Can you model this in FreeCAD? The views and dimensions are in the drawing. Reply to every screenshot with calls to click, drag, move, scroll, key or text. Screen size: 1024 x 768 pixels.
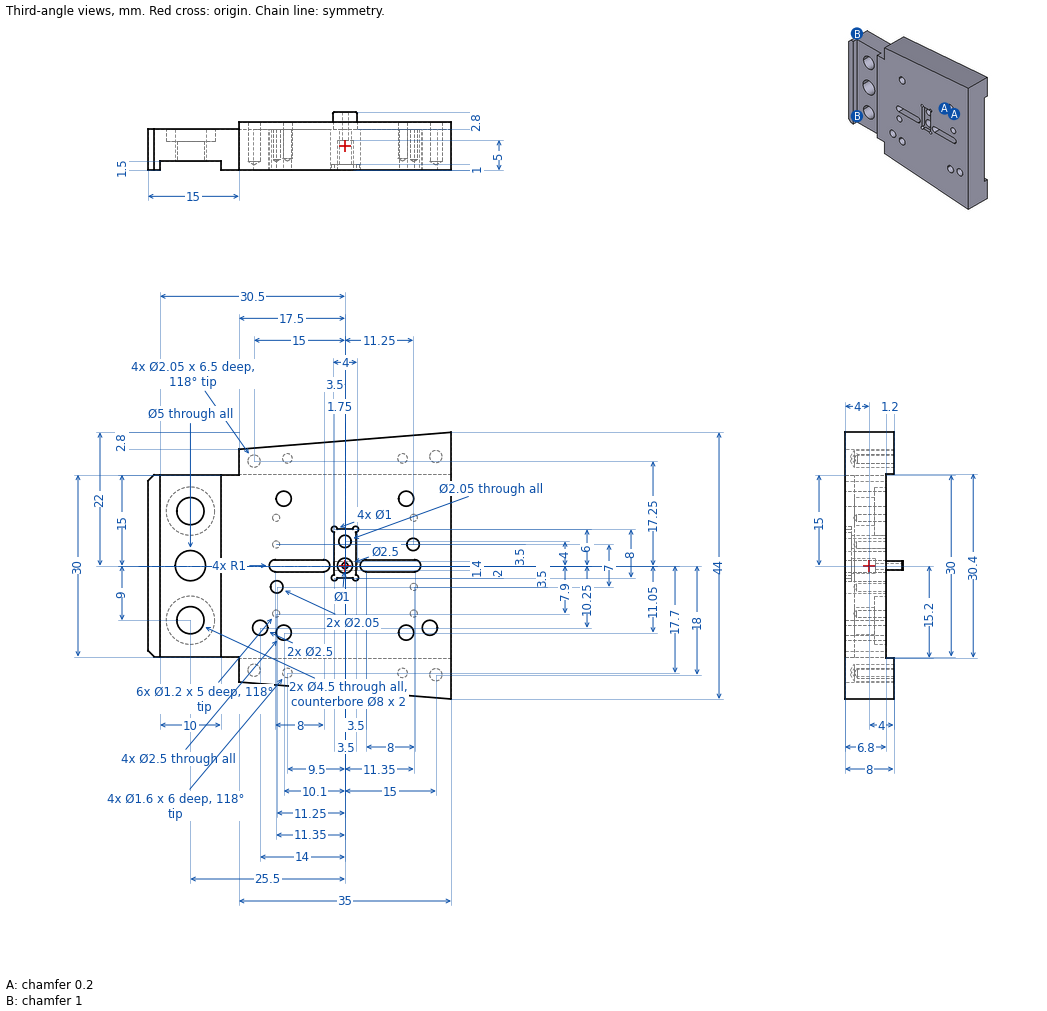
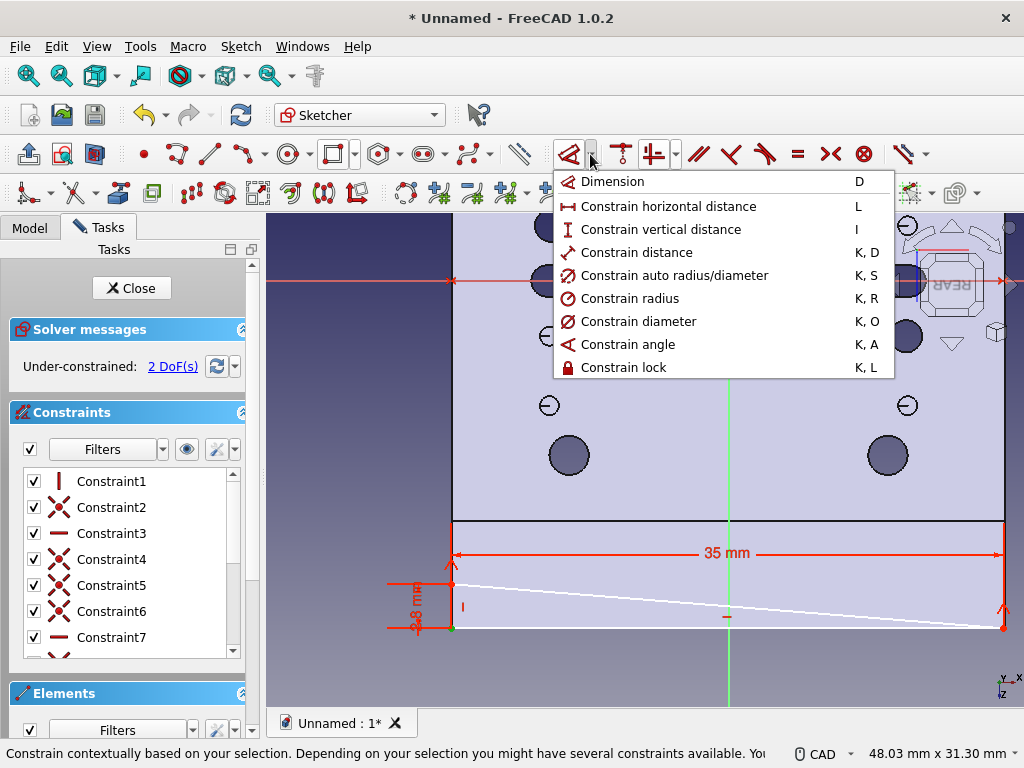
click(724, 230)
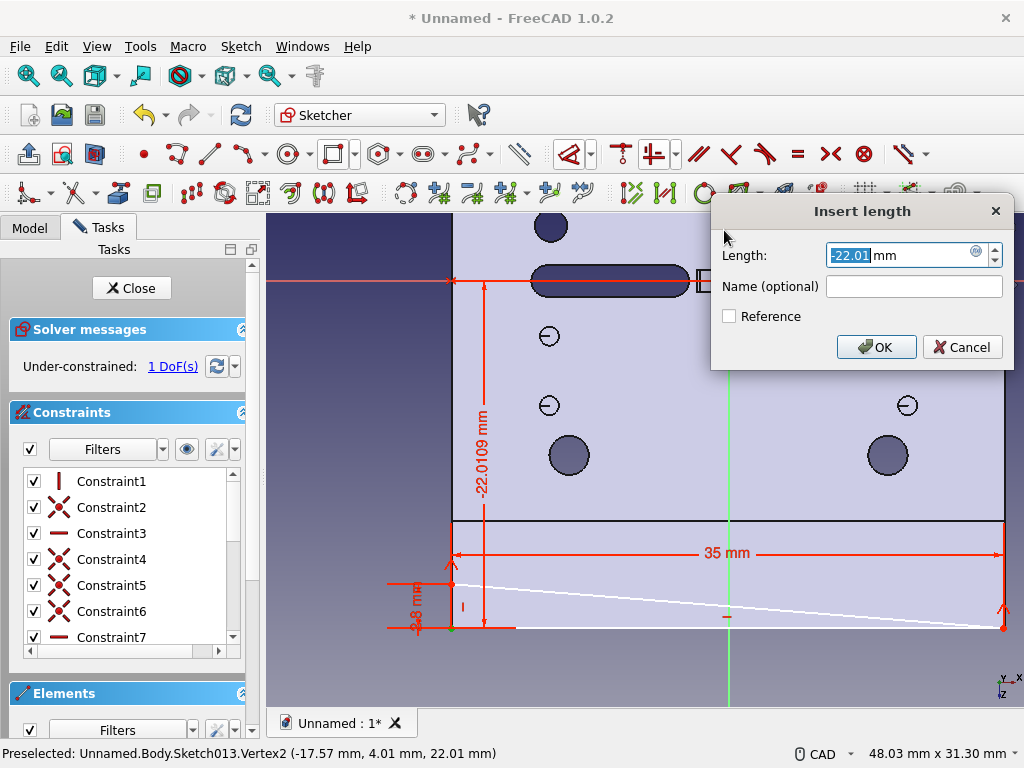
text(-22)
key(Return)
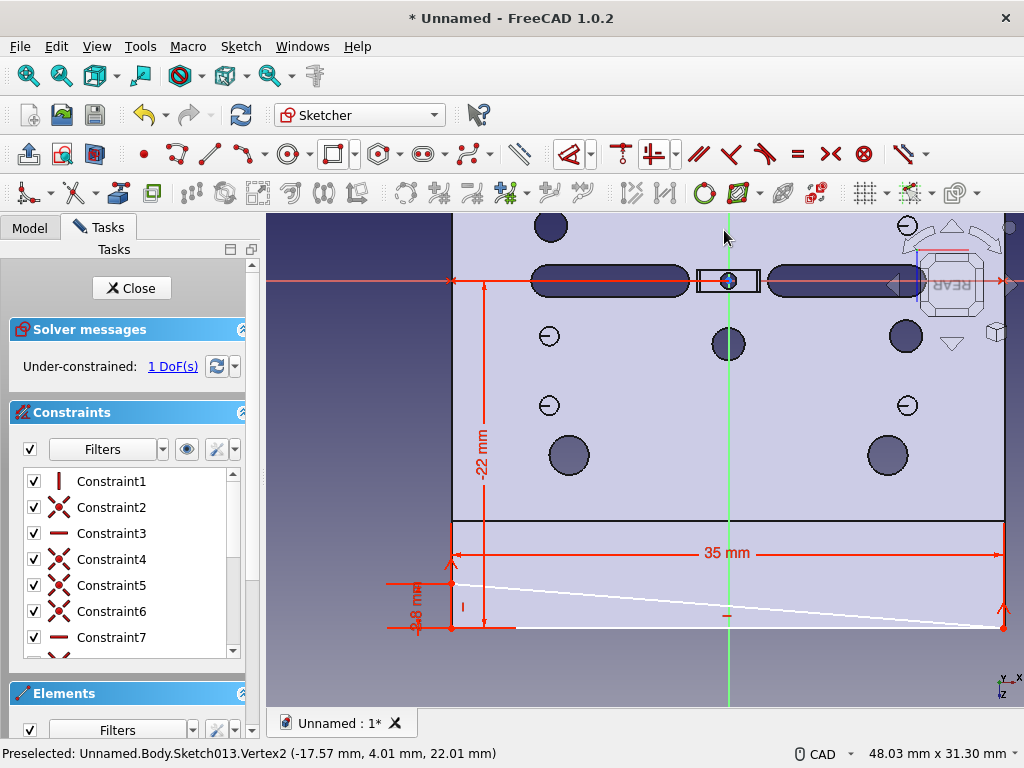
click(451, 584)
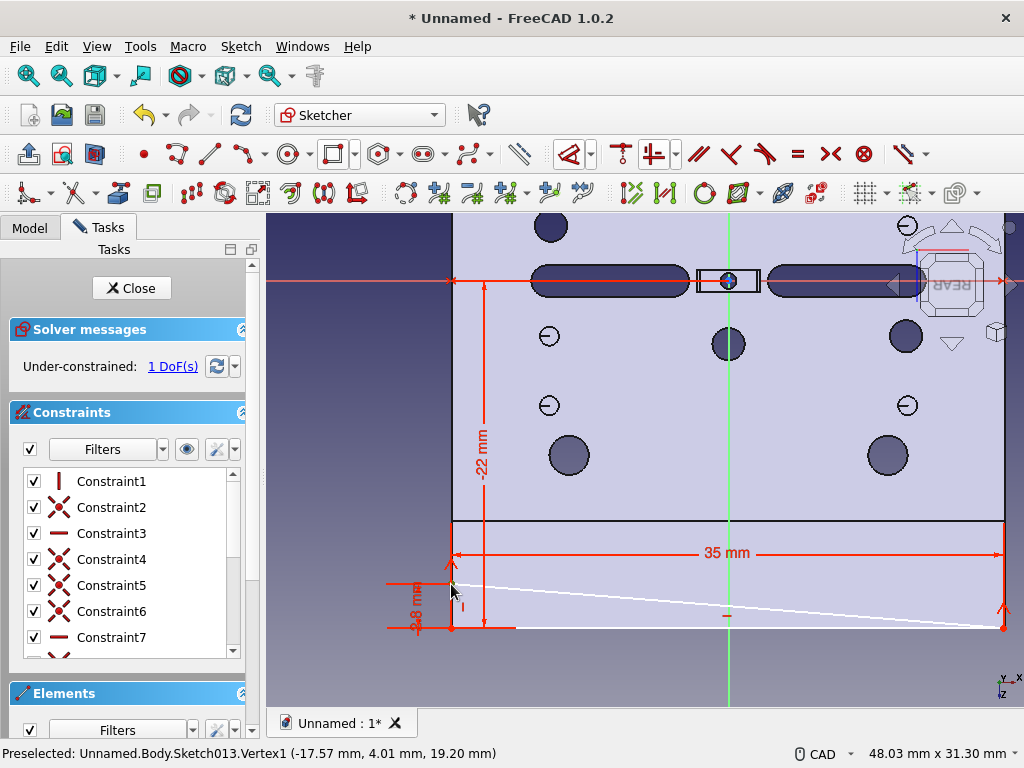
click(590, 154)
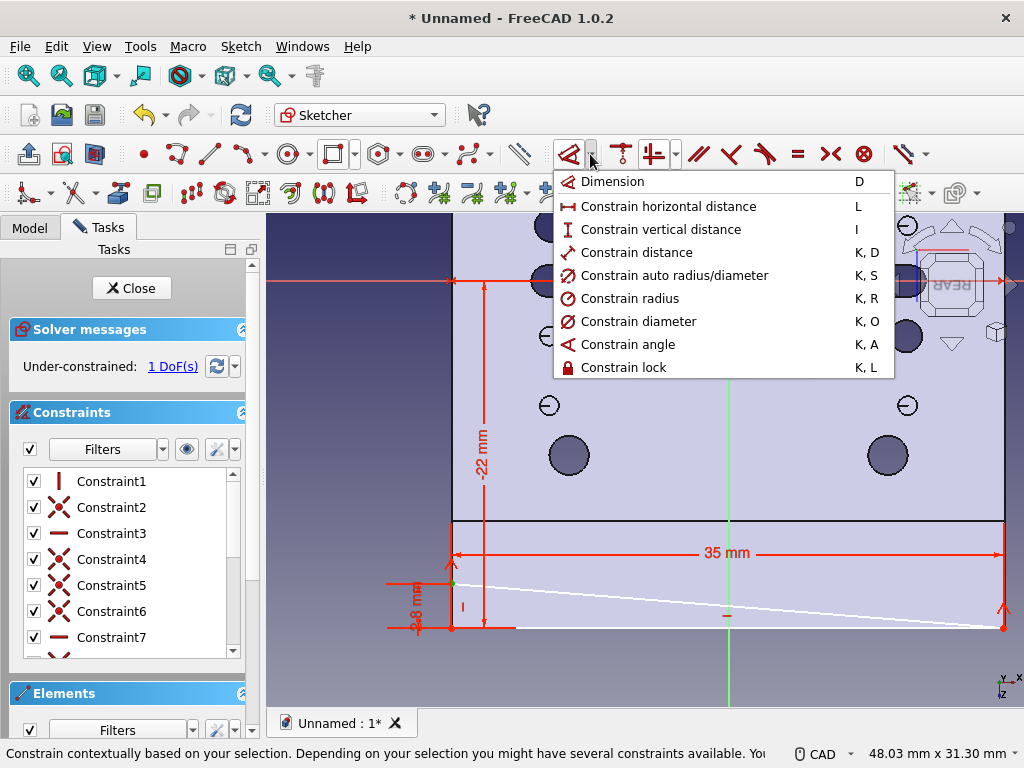
click(724, 206)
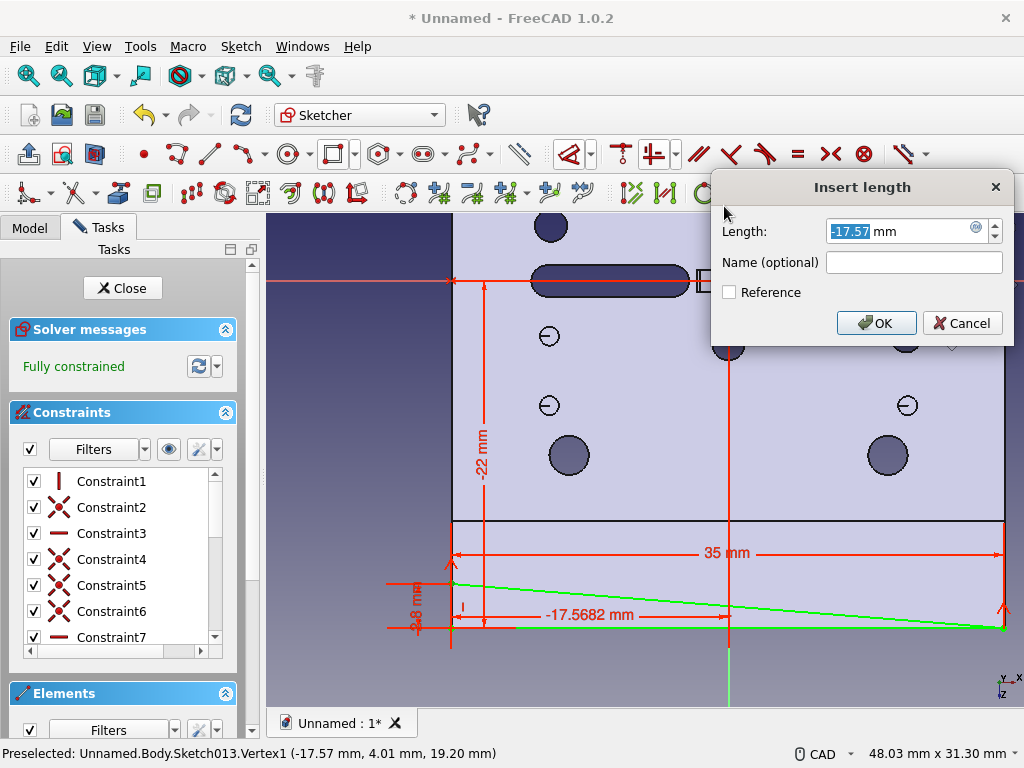
text(-17.5)
key(Return)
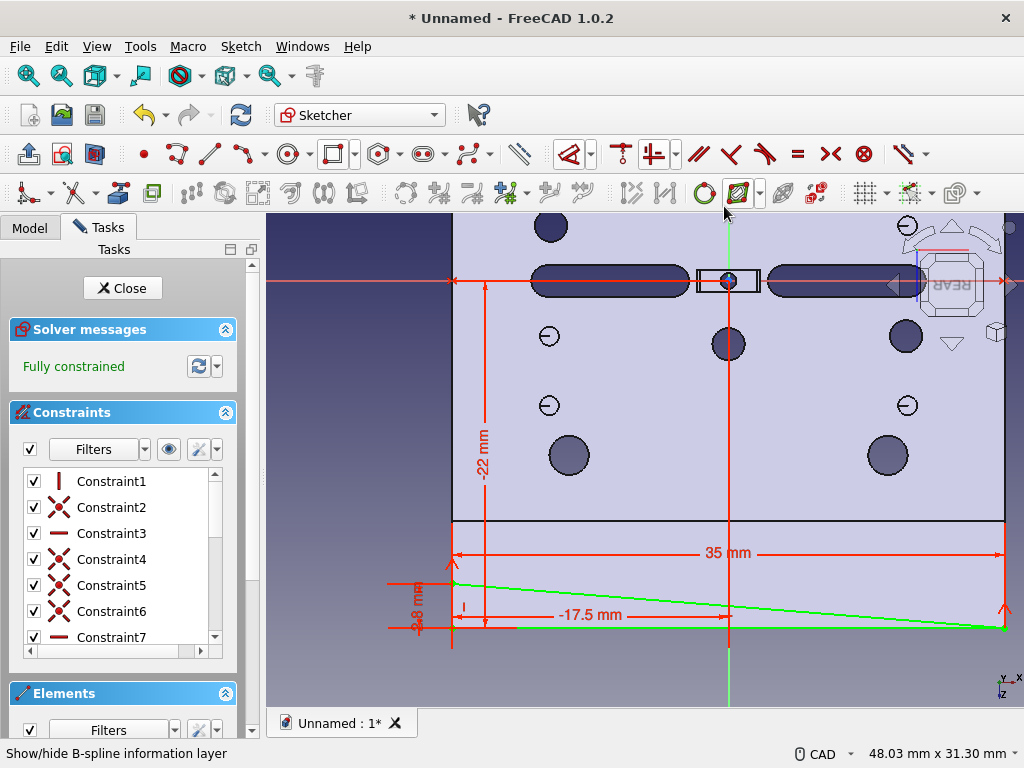
click(123, 288)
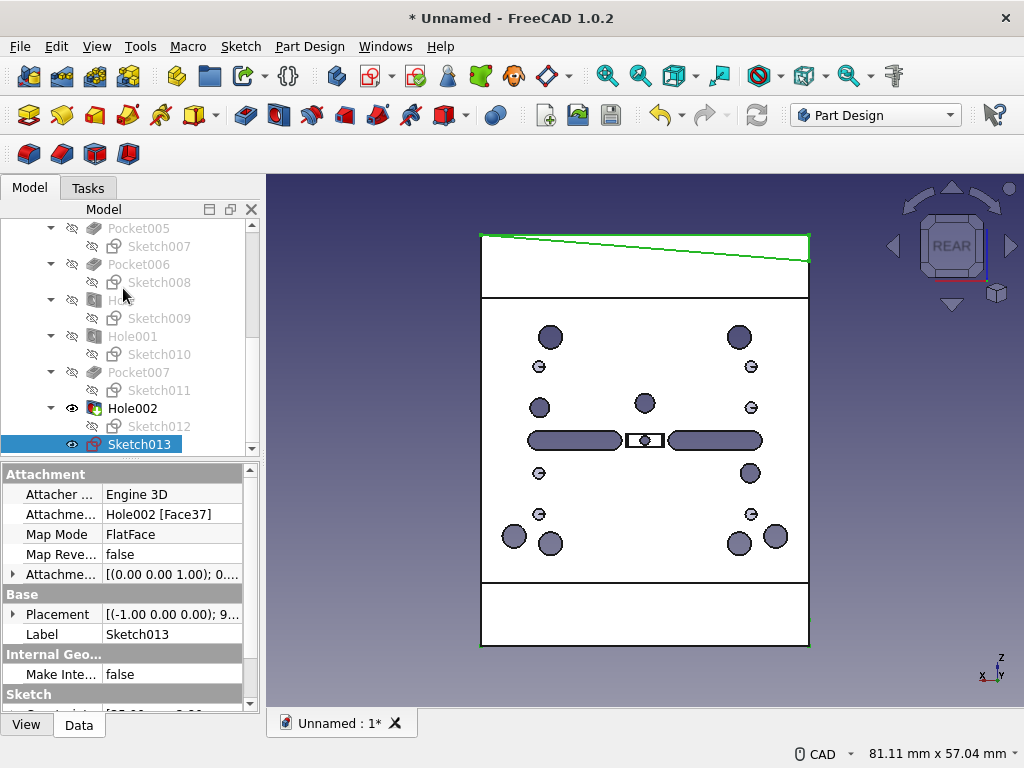
click(246, 116)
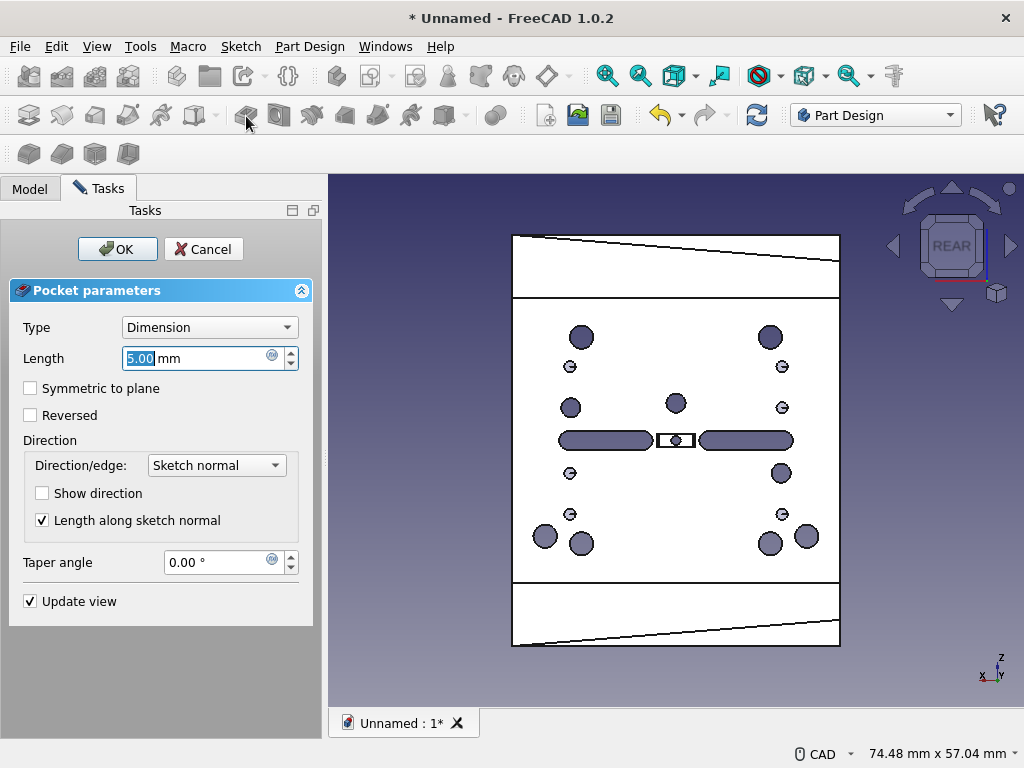
click(210, 328)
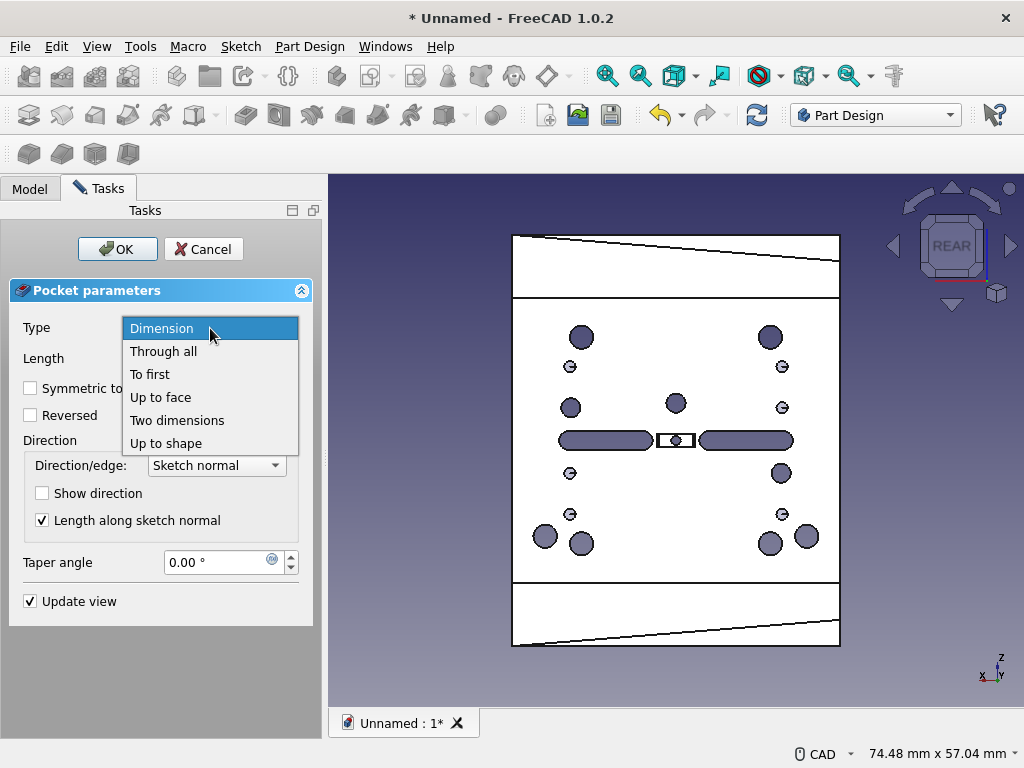
click(208, 352)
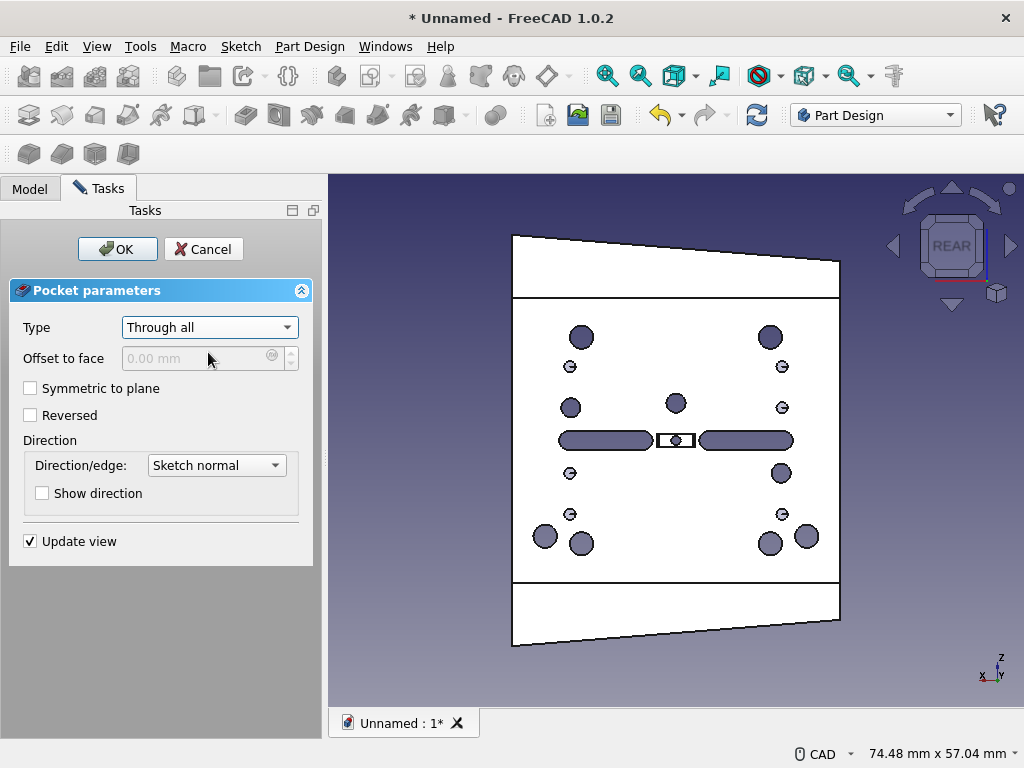
click(118, 249)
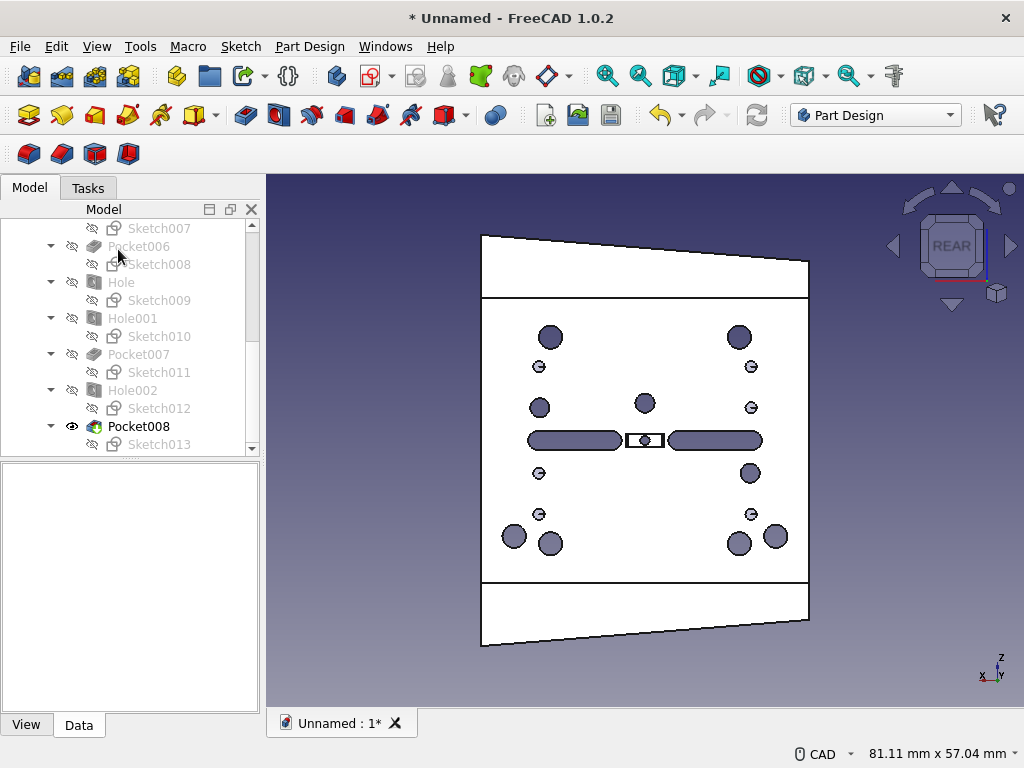
click(552, 613)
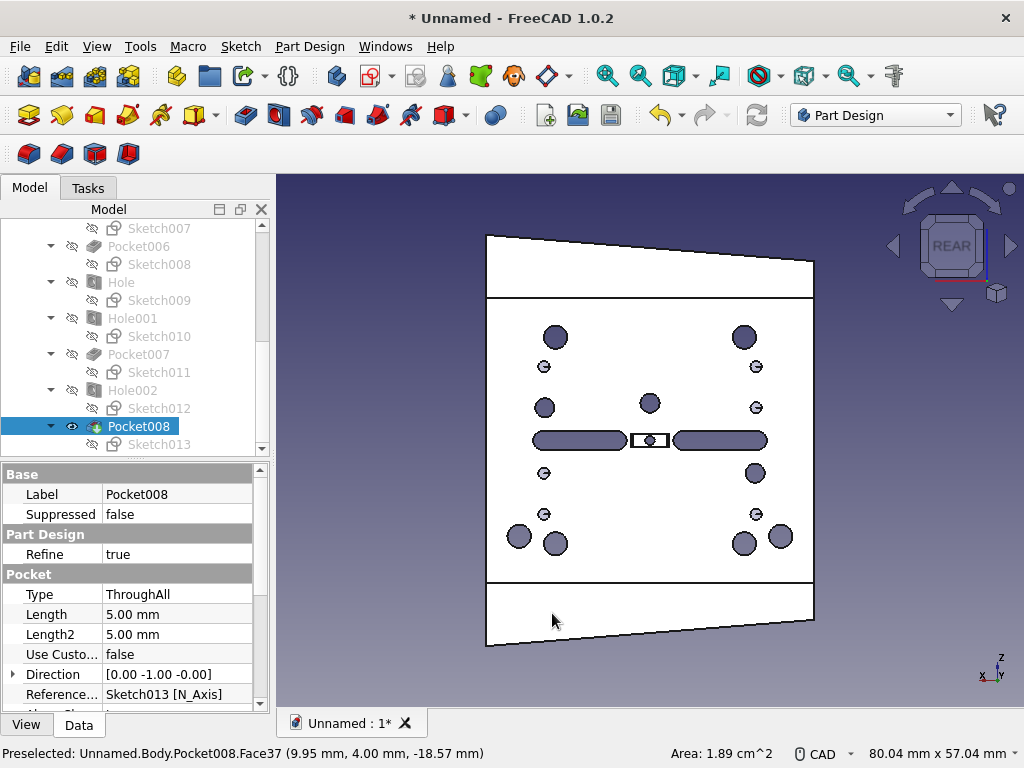
click(370, 76)